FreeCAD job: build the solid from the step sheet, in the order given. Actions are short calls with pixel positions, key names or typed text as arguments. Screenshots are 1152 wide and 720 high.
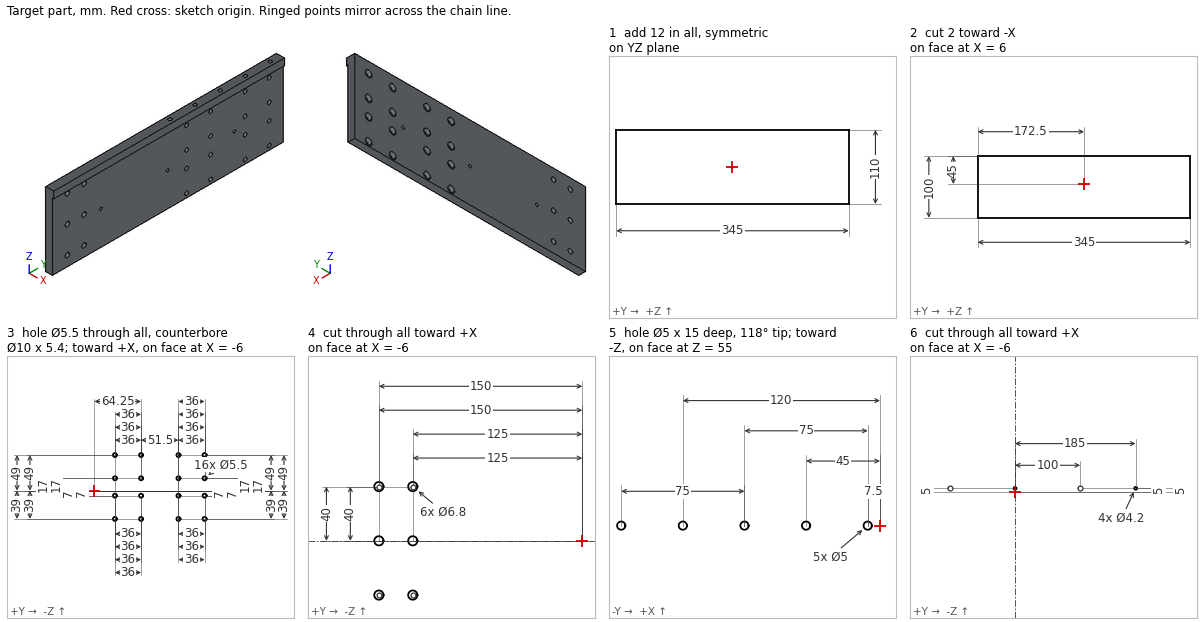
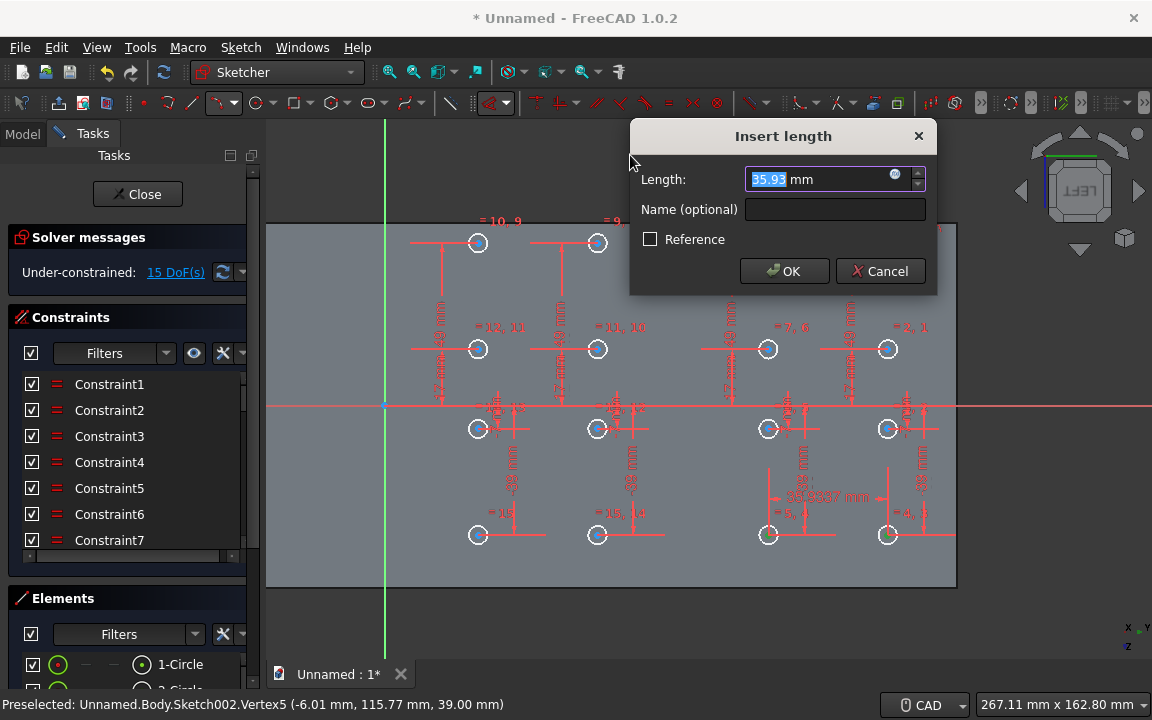
text(36)
key(Return)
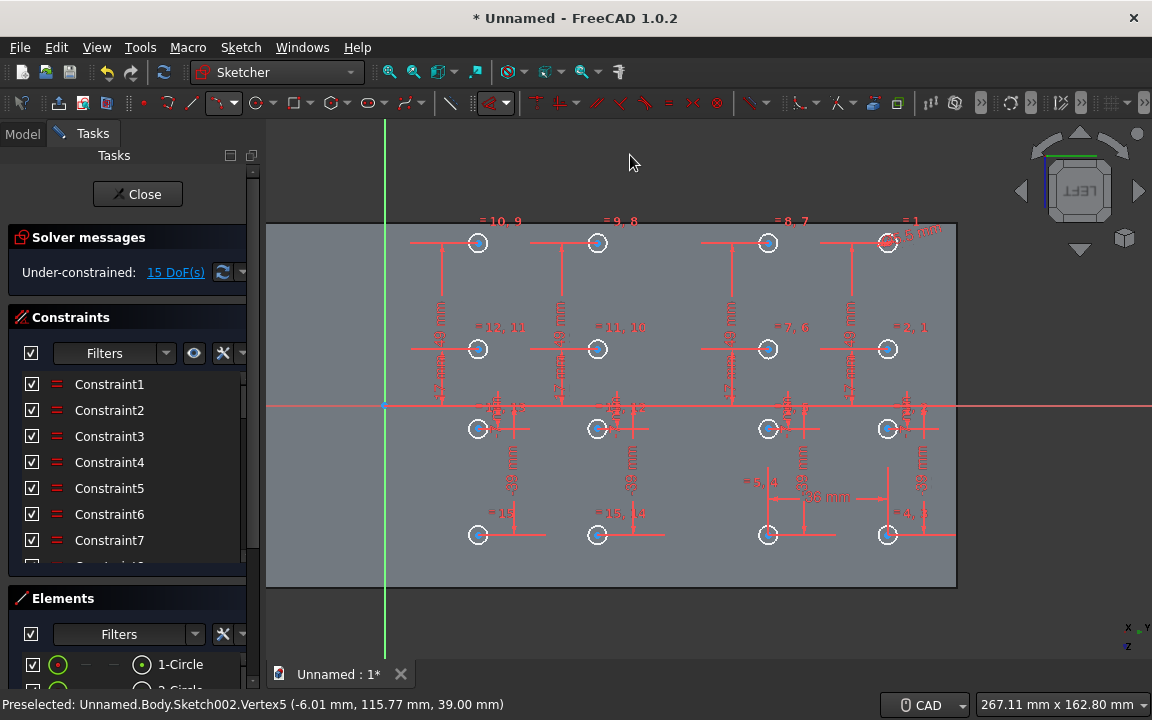
click(888, 429)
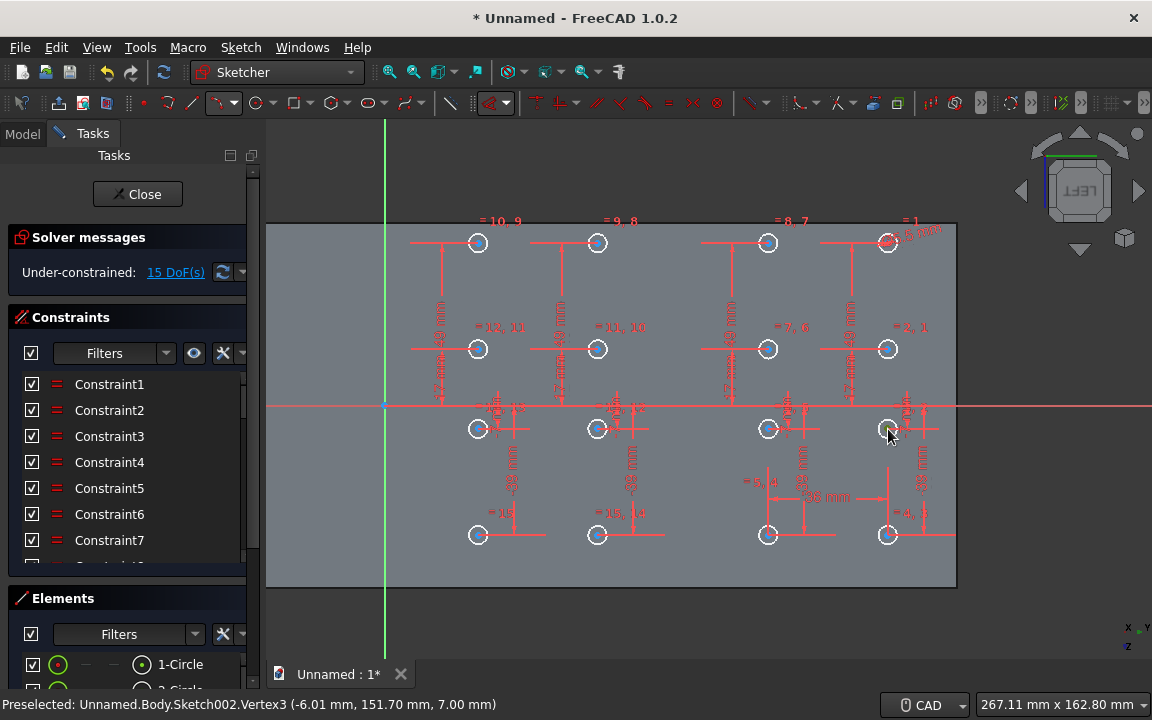
click(768, 535)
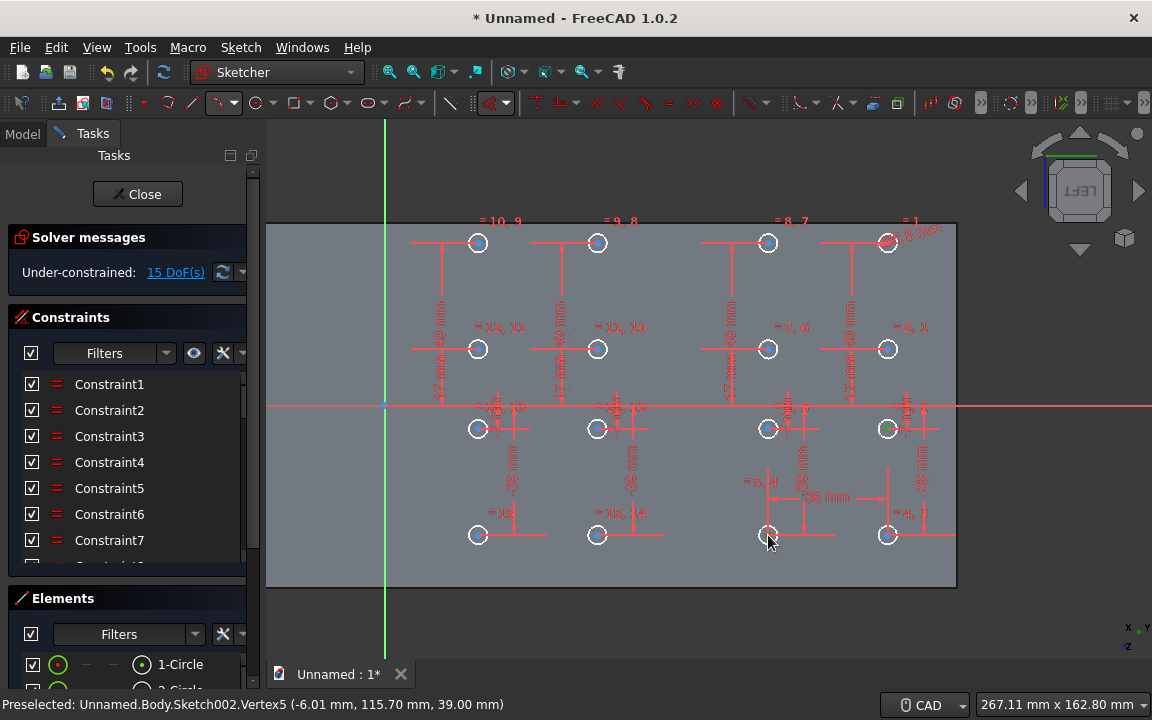
click(508, 104)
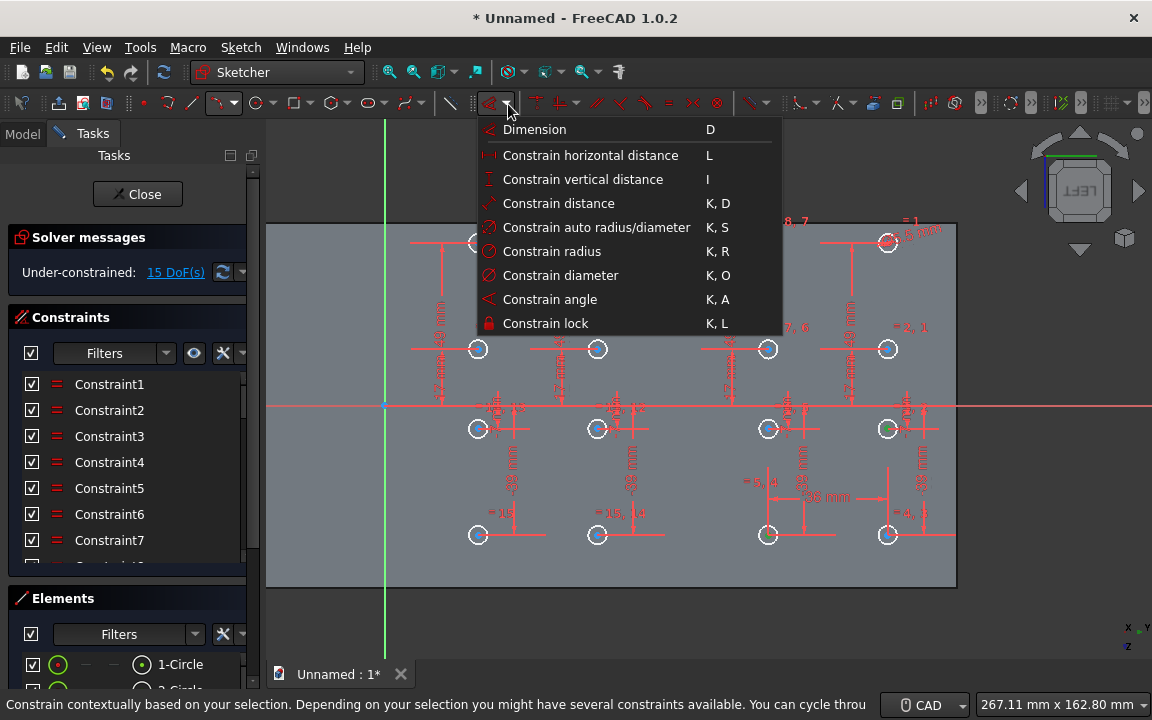
click(630, 155)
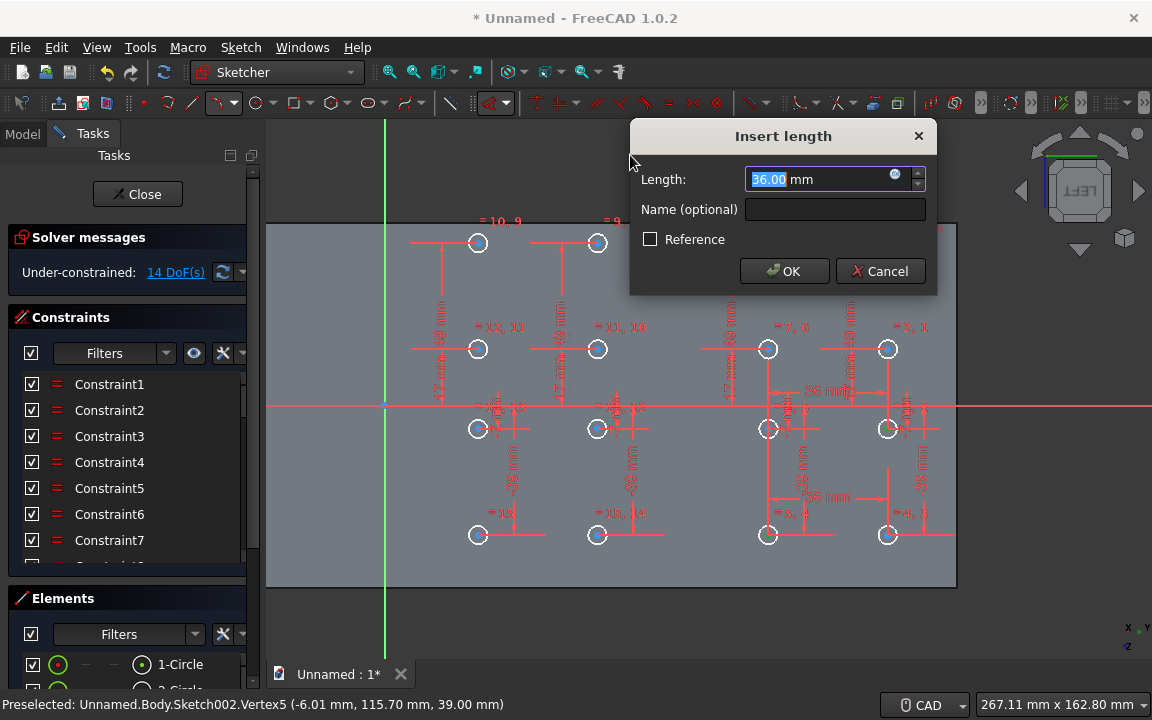
text(36)
key(Return)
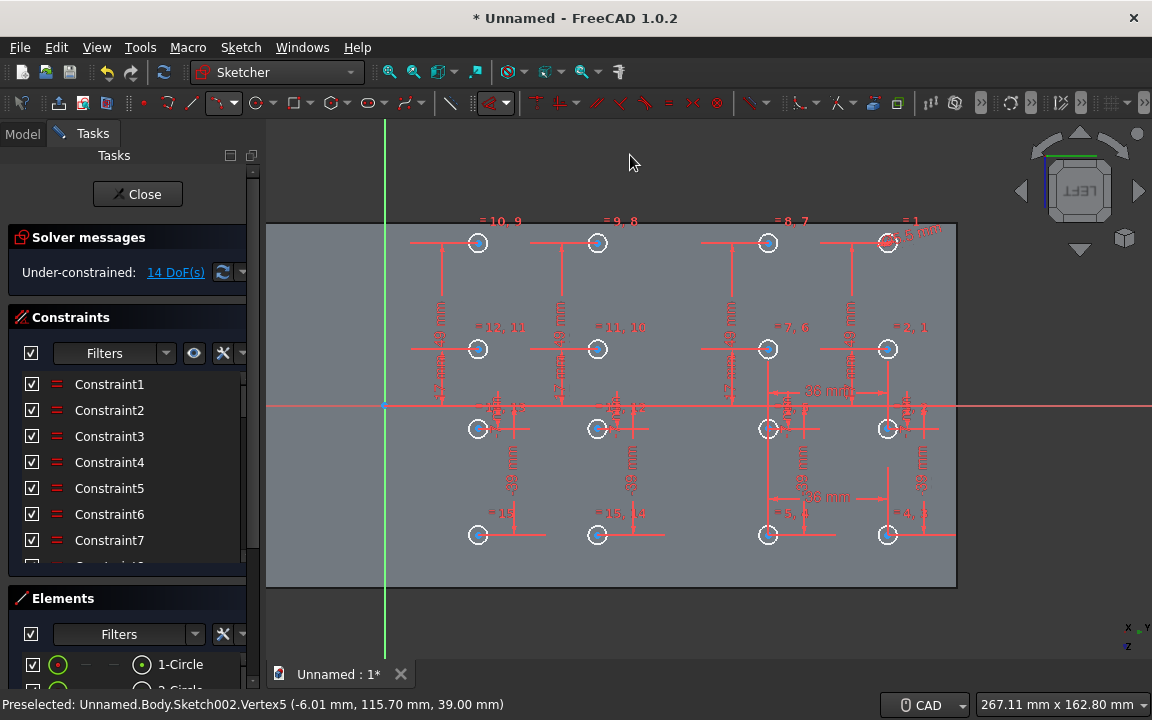
click(888, 349)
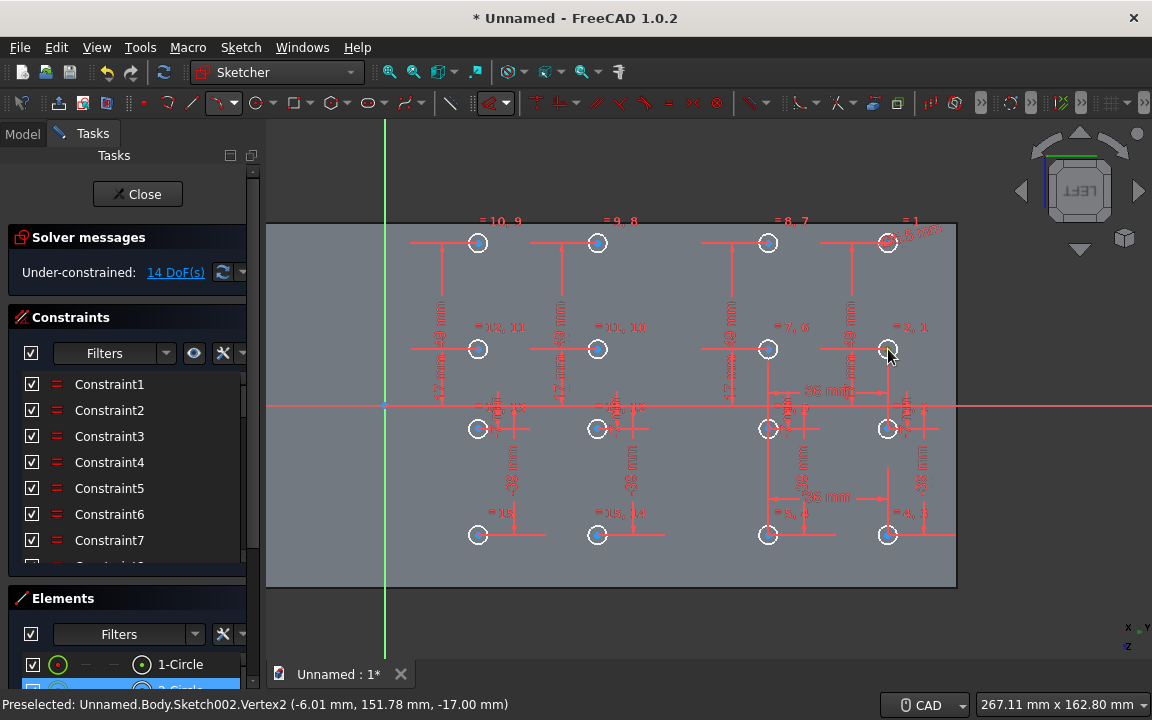
click(768, 535)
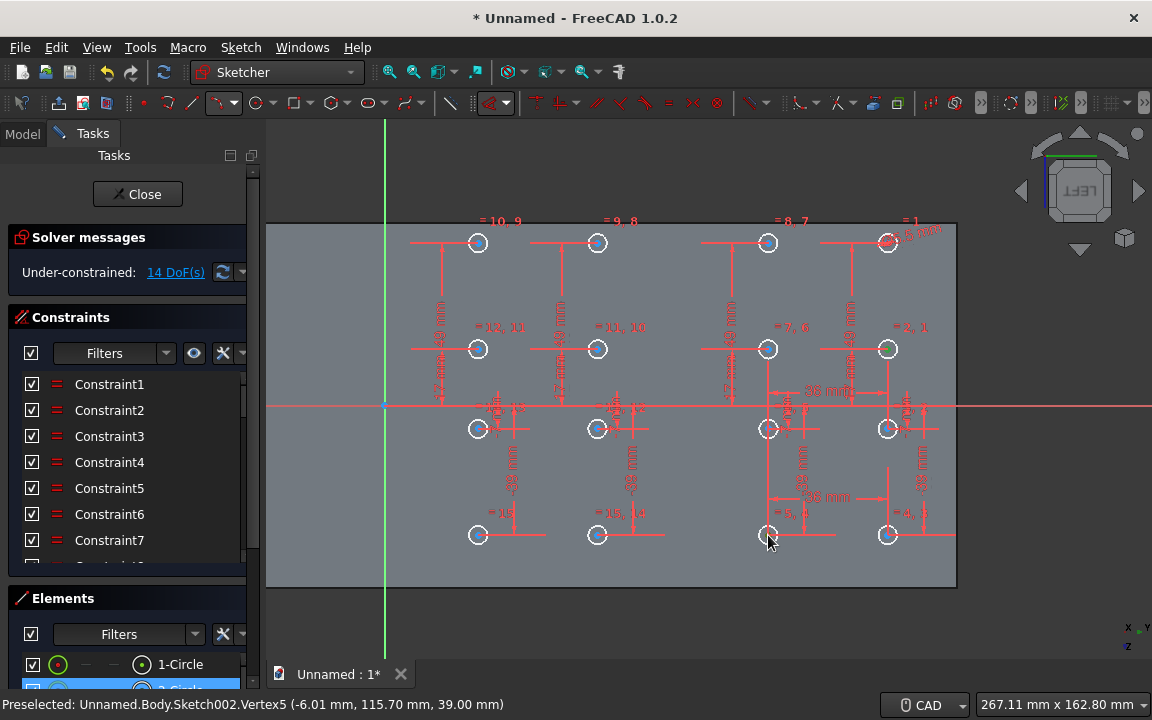
click(508, 104)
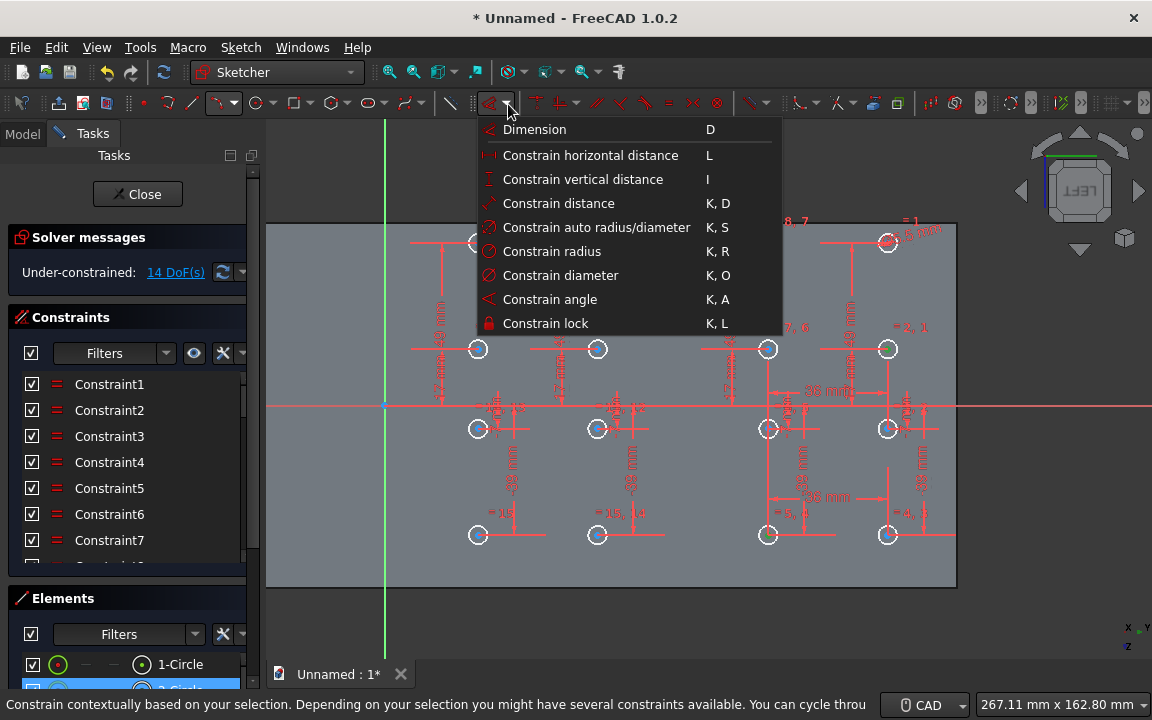
click(630, 155)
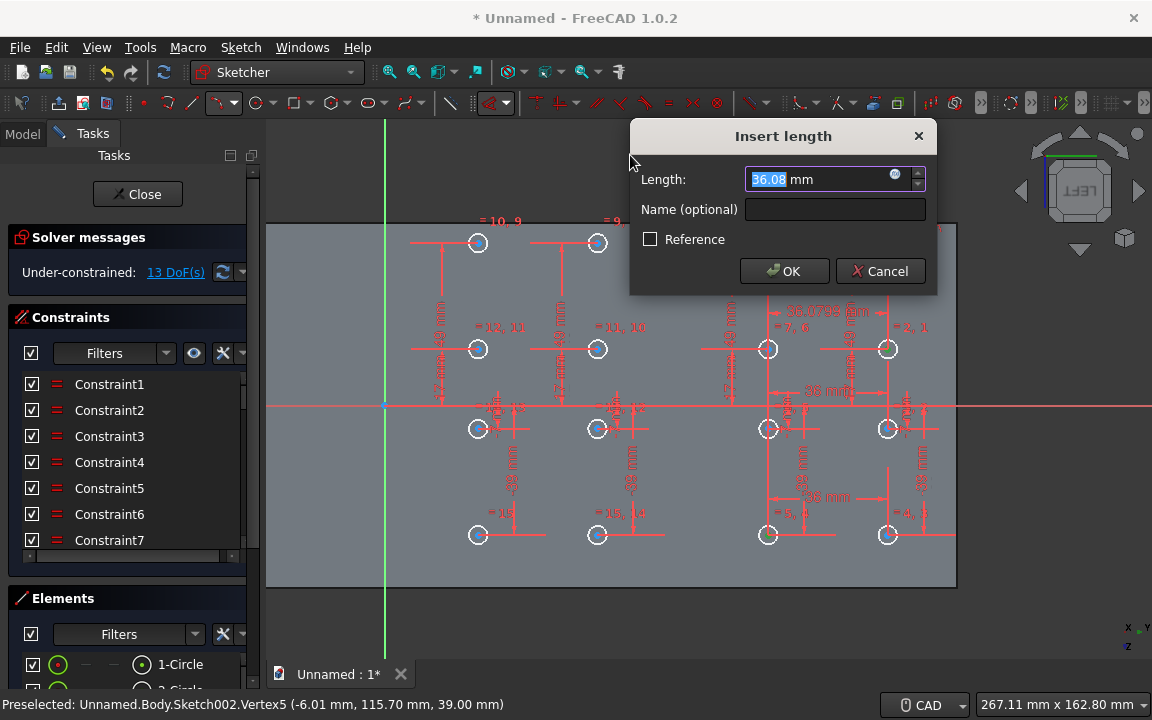
text(36)
key(Return)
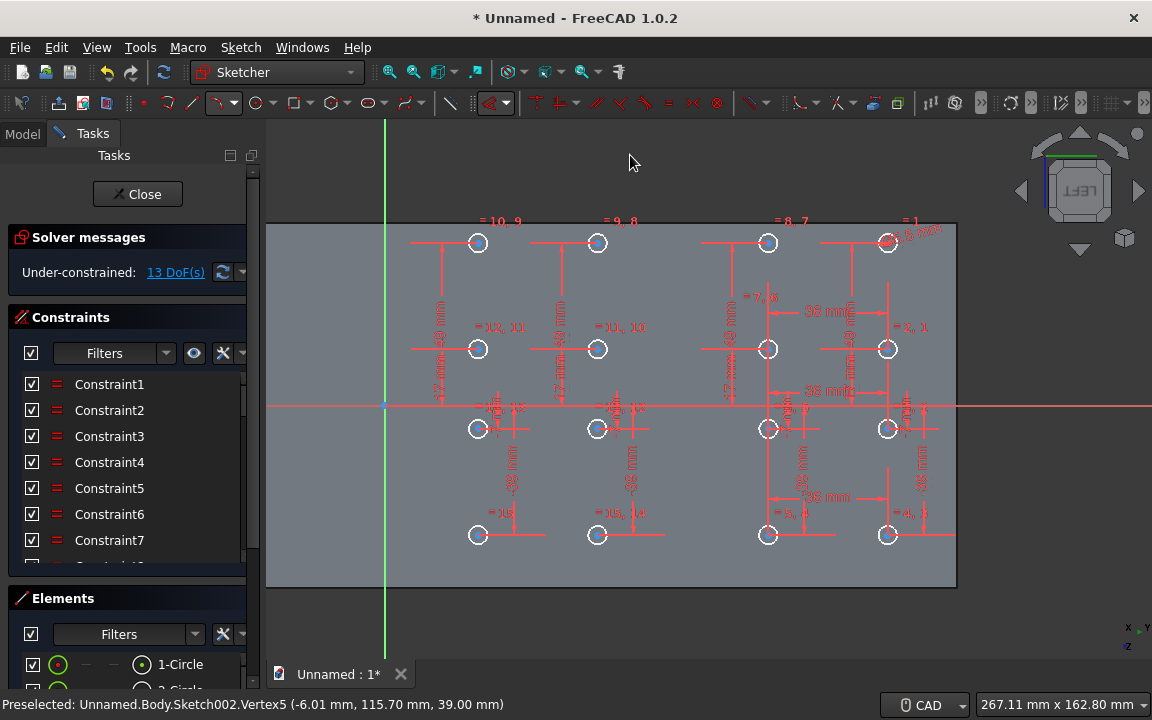
click(888, 243)